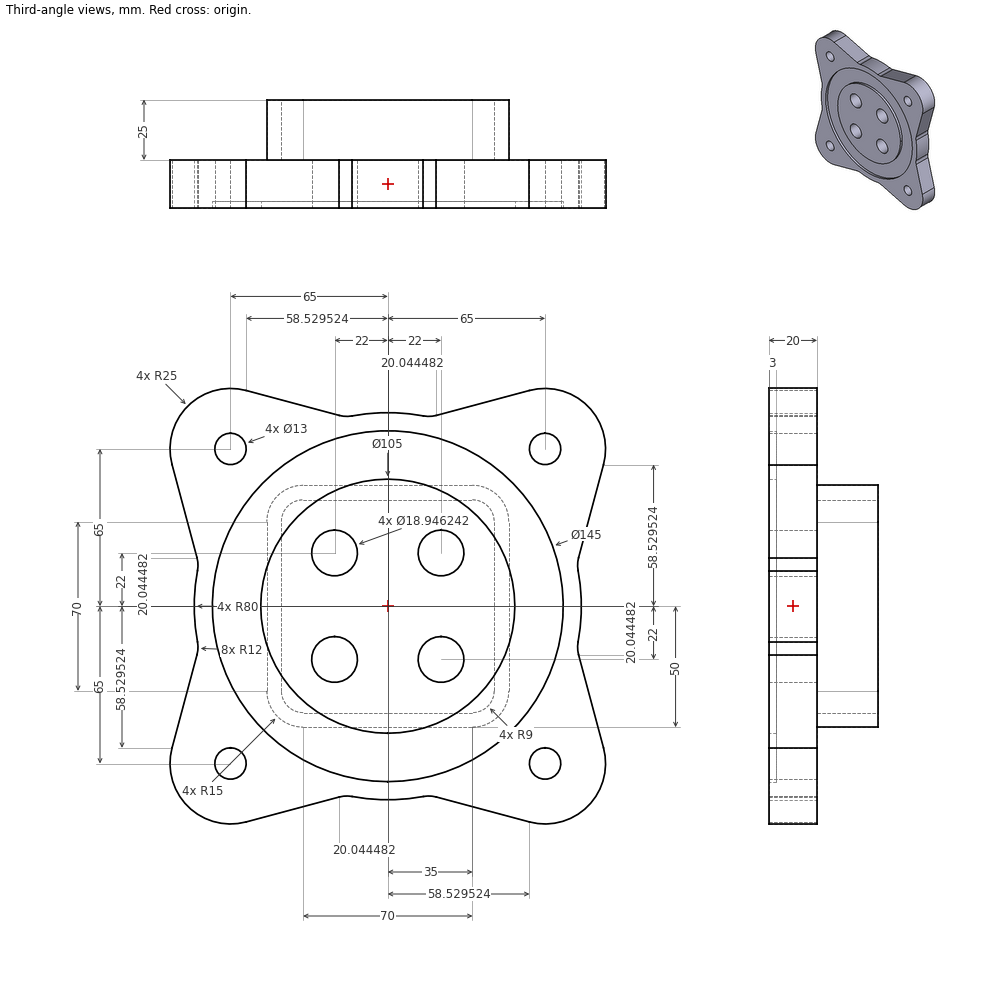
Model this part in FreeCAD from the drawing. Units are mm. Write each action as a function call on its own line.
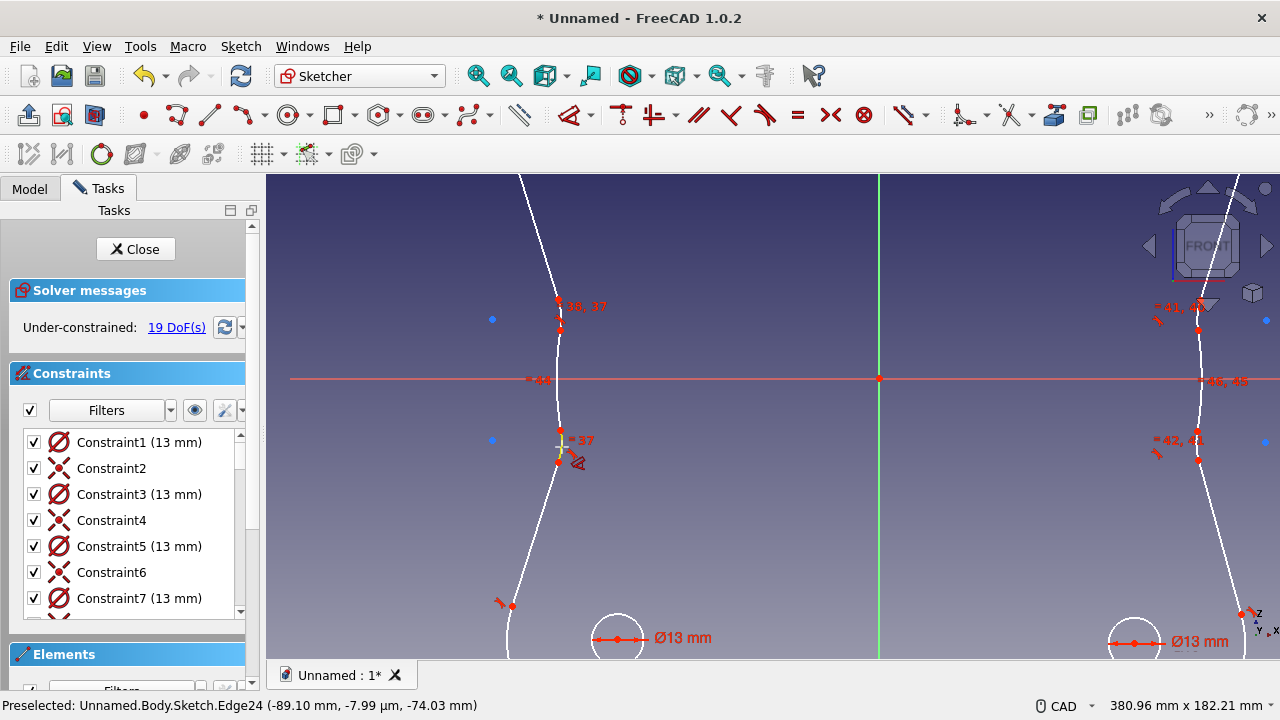
click(562, 446)
click(594, 448)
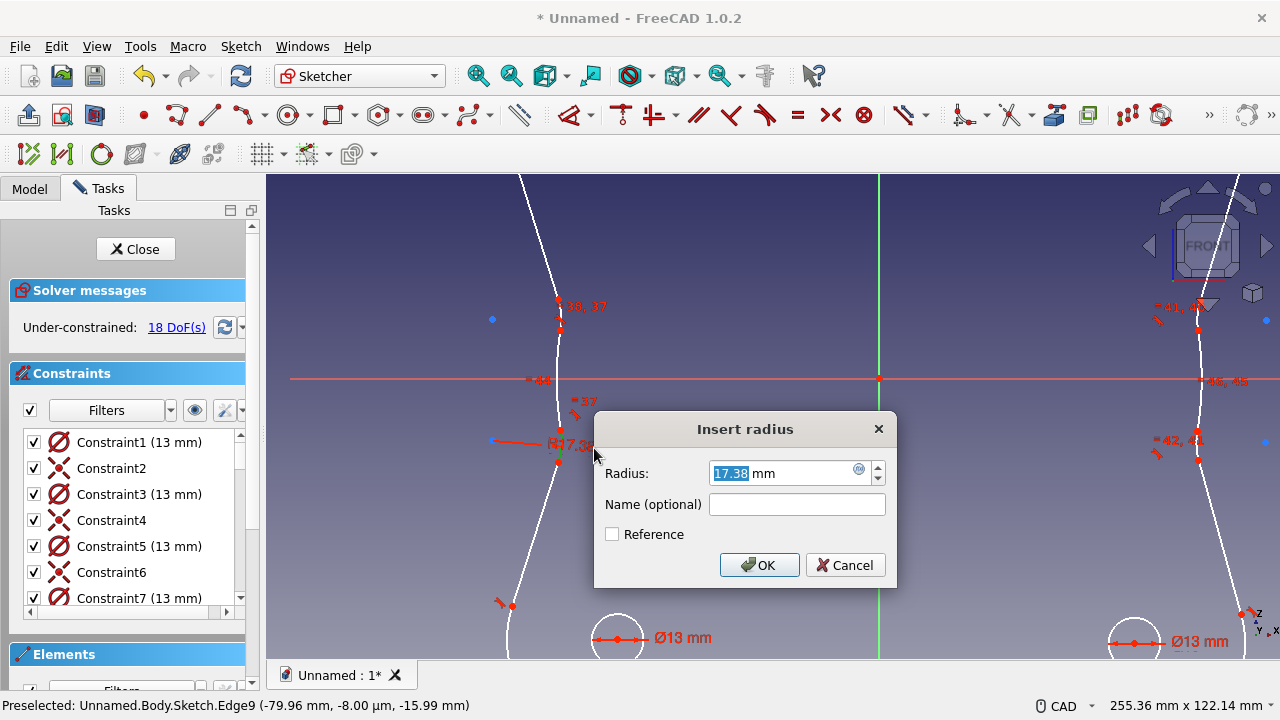
text(12)
key(Return)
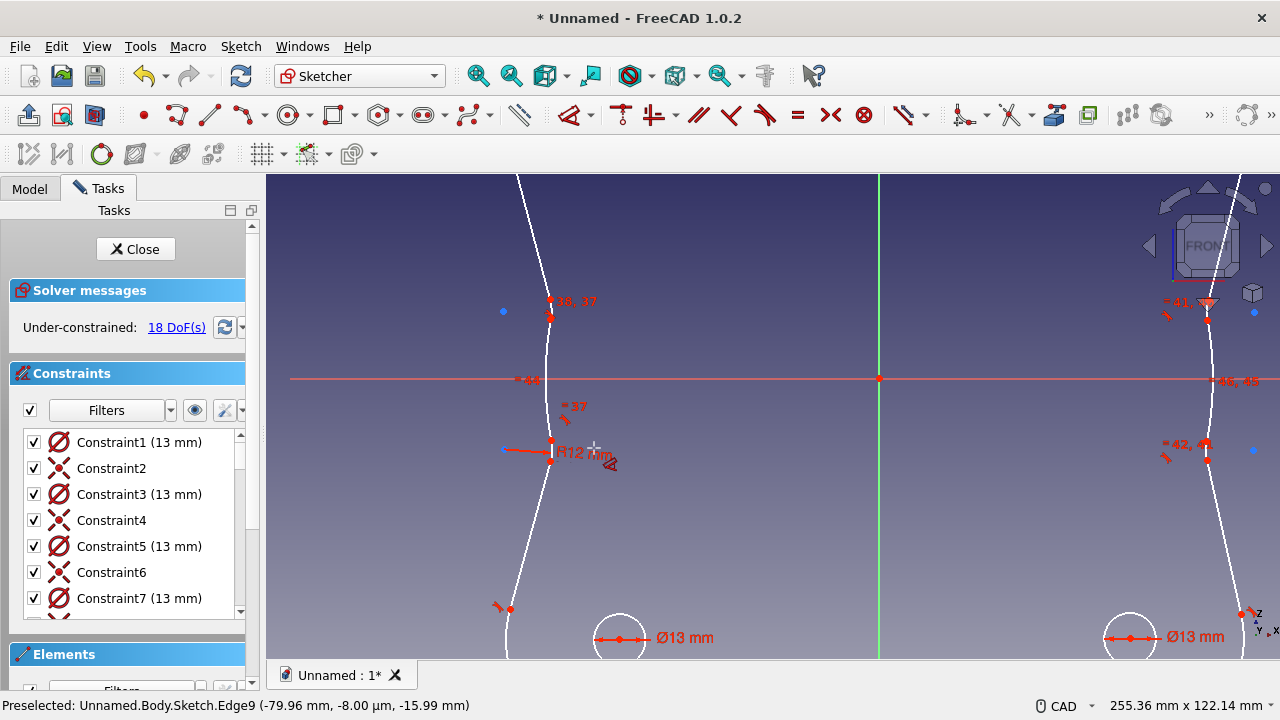
click(546, 356)
click(514, 354)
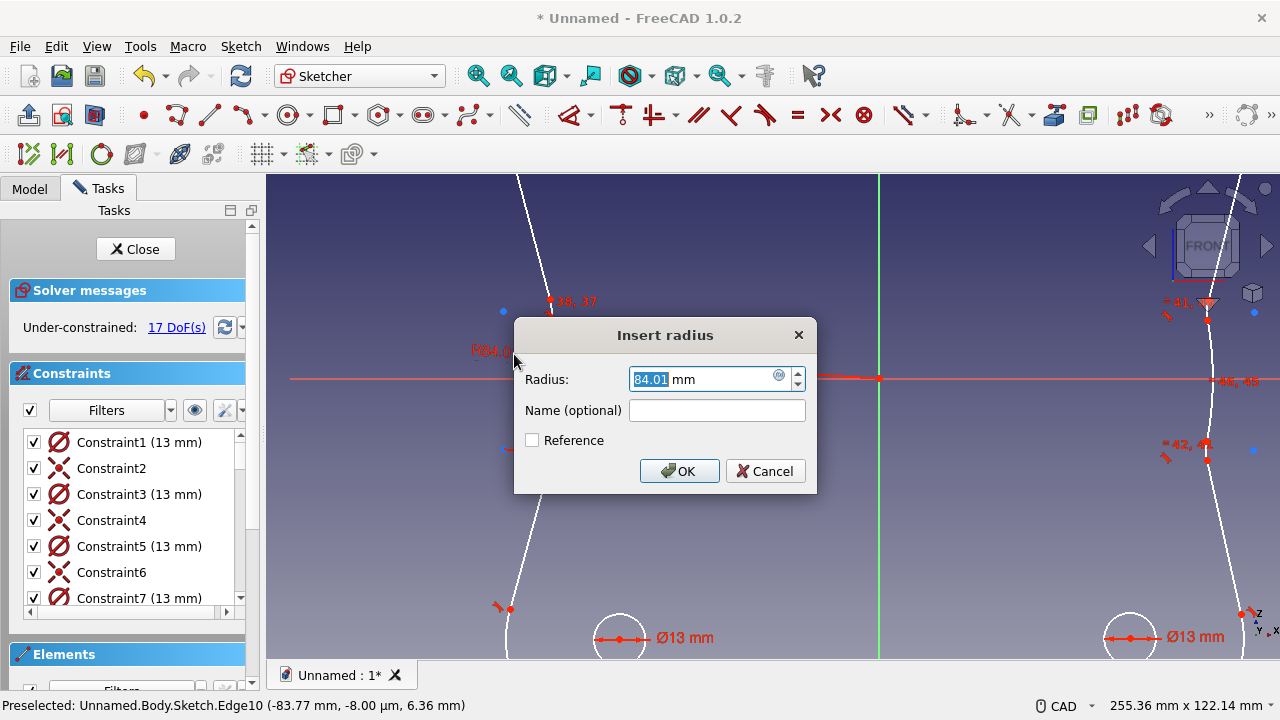
text(80)
key(Return)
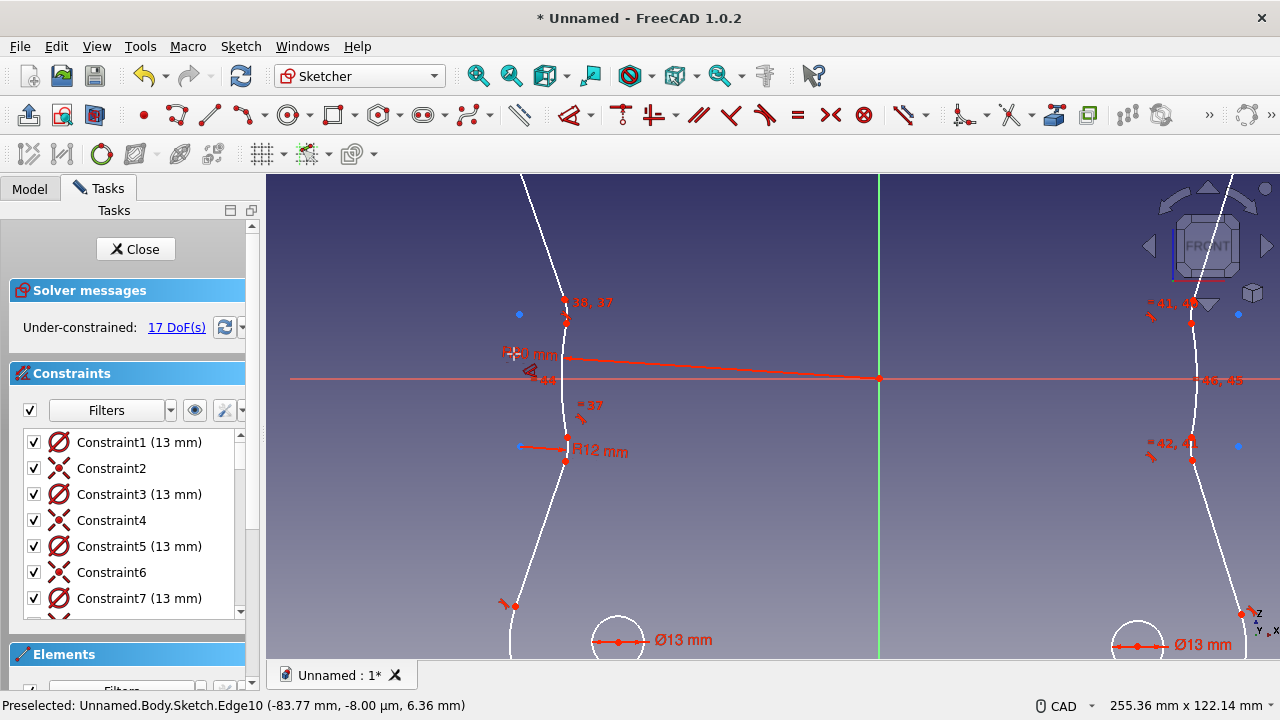
scroll(562, 447, down, 4)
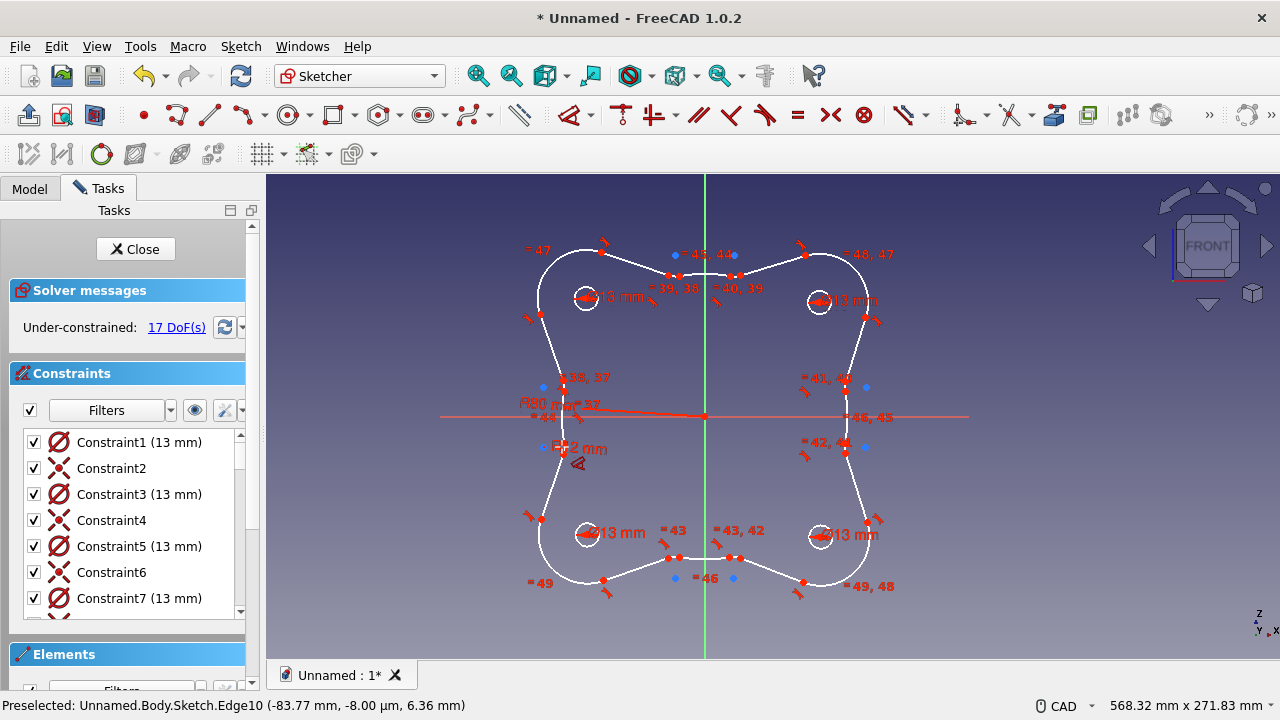
click(570, 253)
click(559, 223)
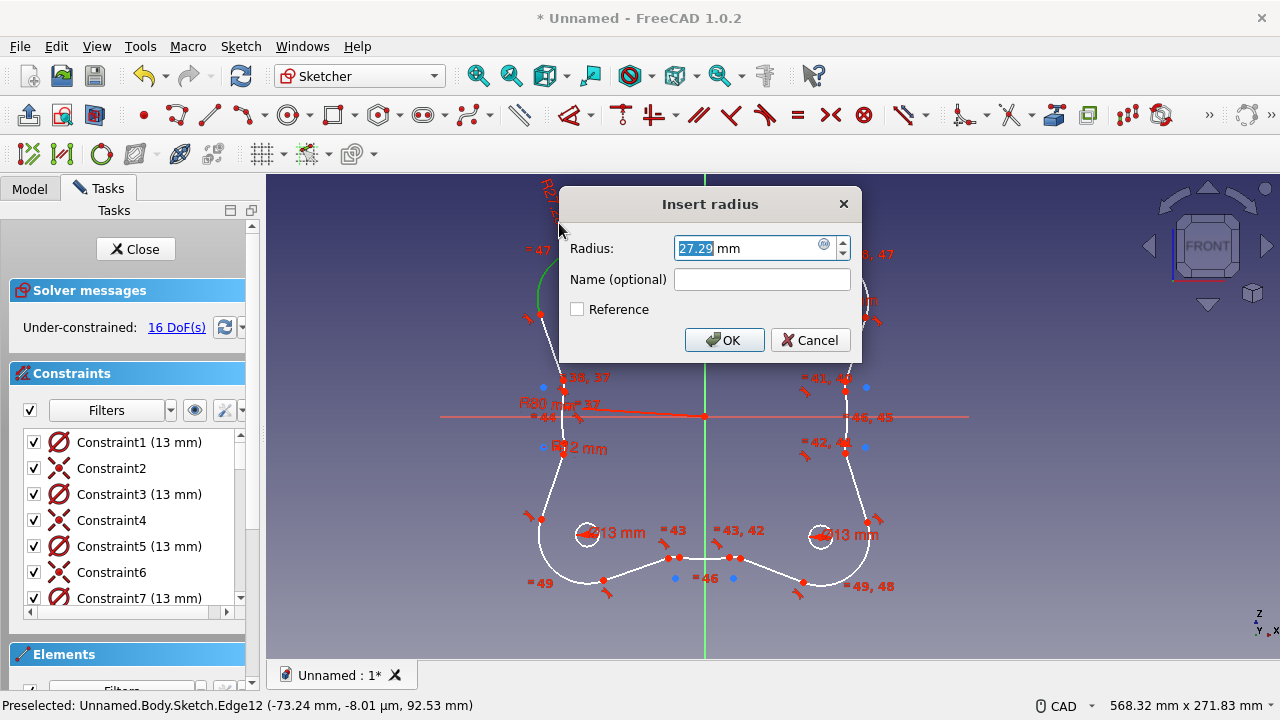
text(25)
key(Return)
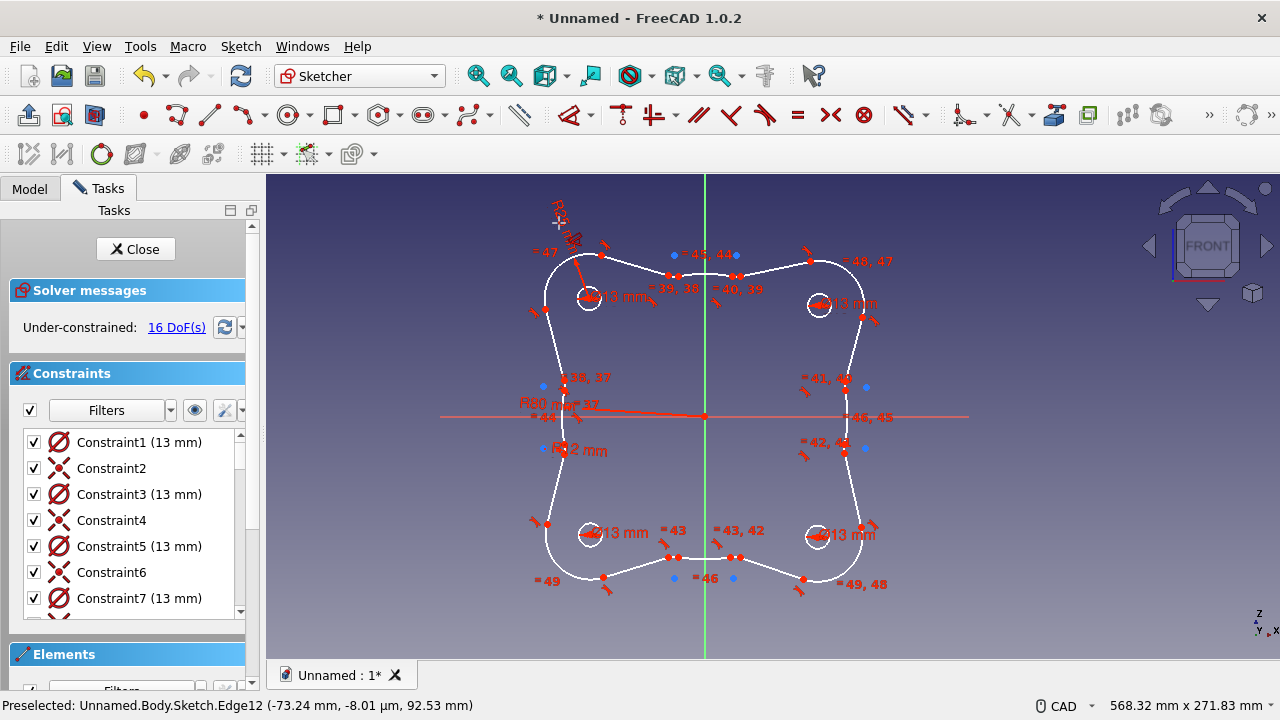
click(589, 299)
click(647, 451)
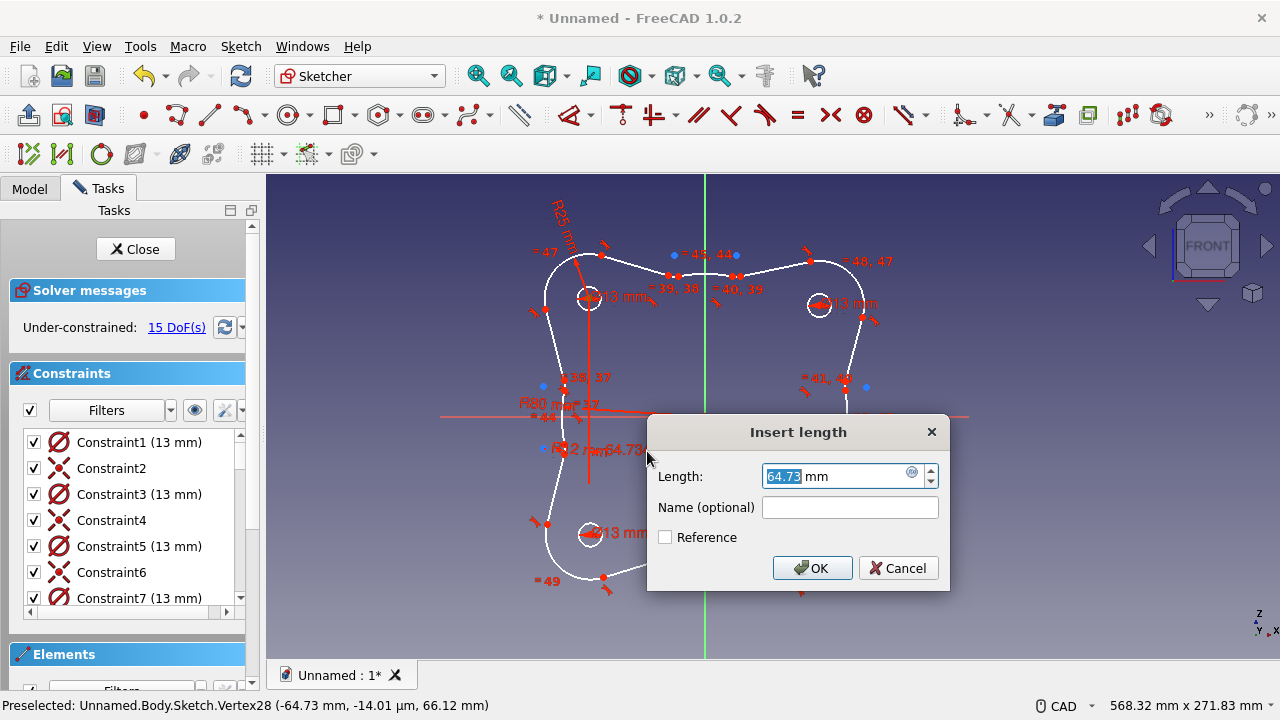
text(65)
key(Return)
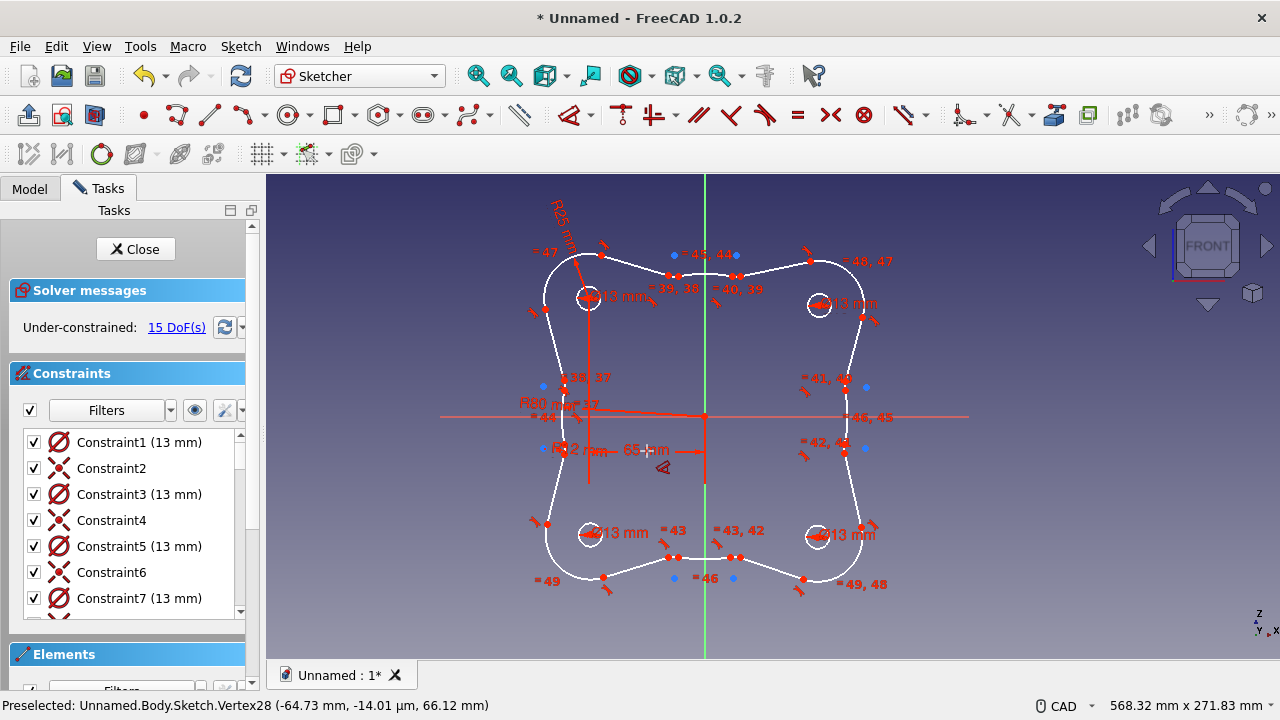
click(589, 298)
click(739, 358)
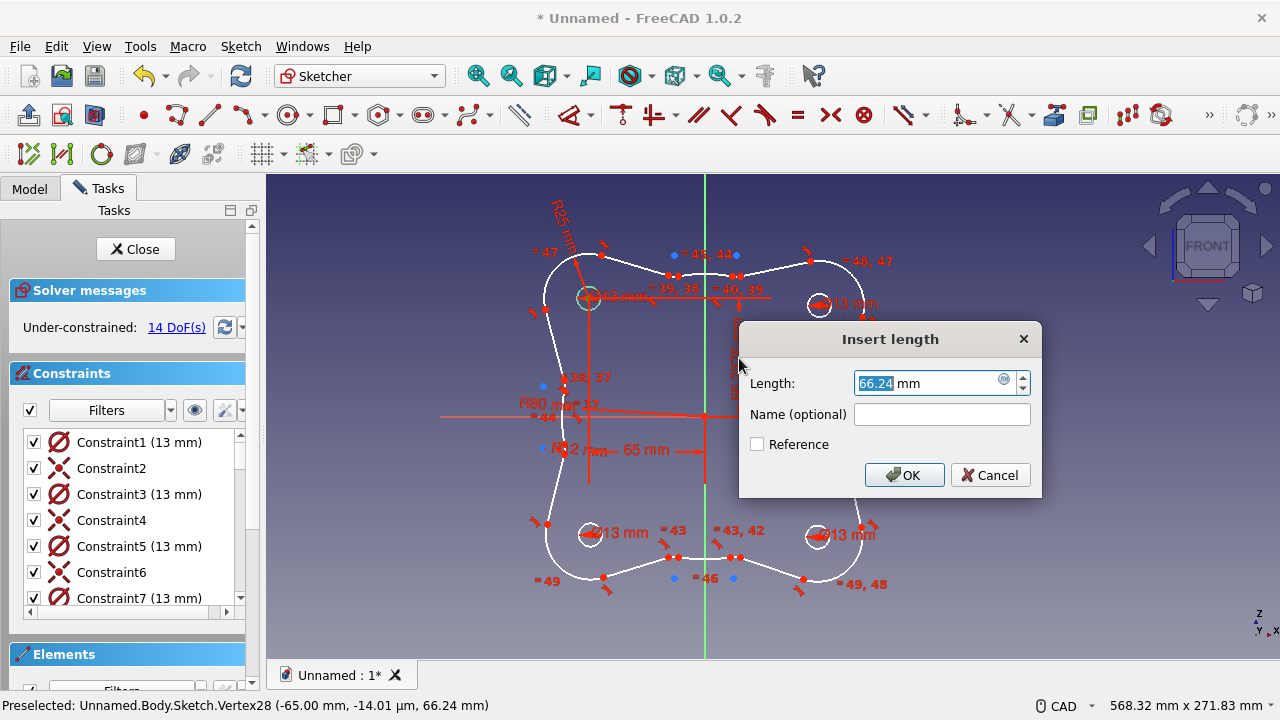
text(65)
key(Return)